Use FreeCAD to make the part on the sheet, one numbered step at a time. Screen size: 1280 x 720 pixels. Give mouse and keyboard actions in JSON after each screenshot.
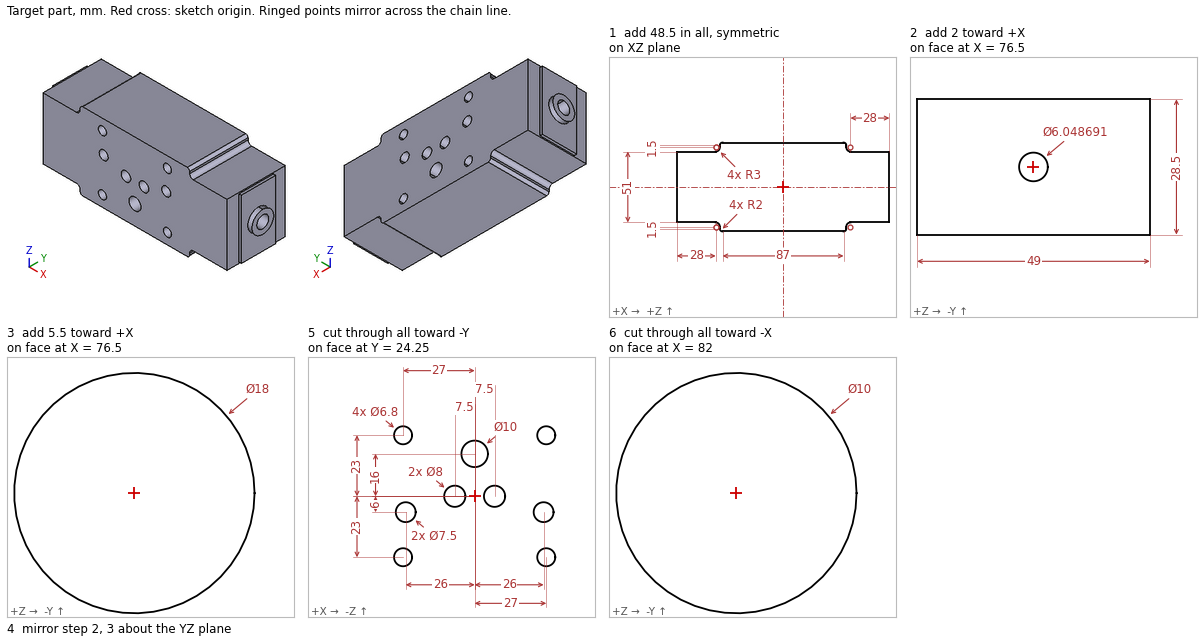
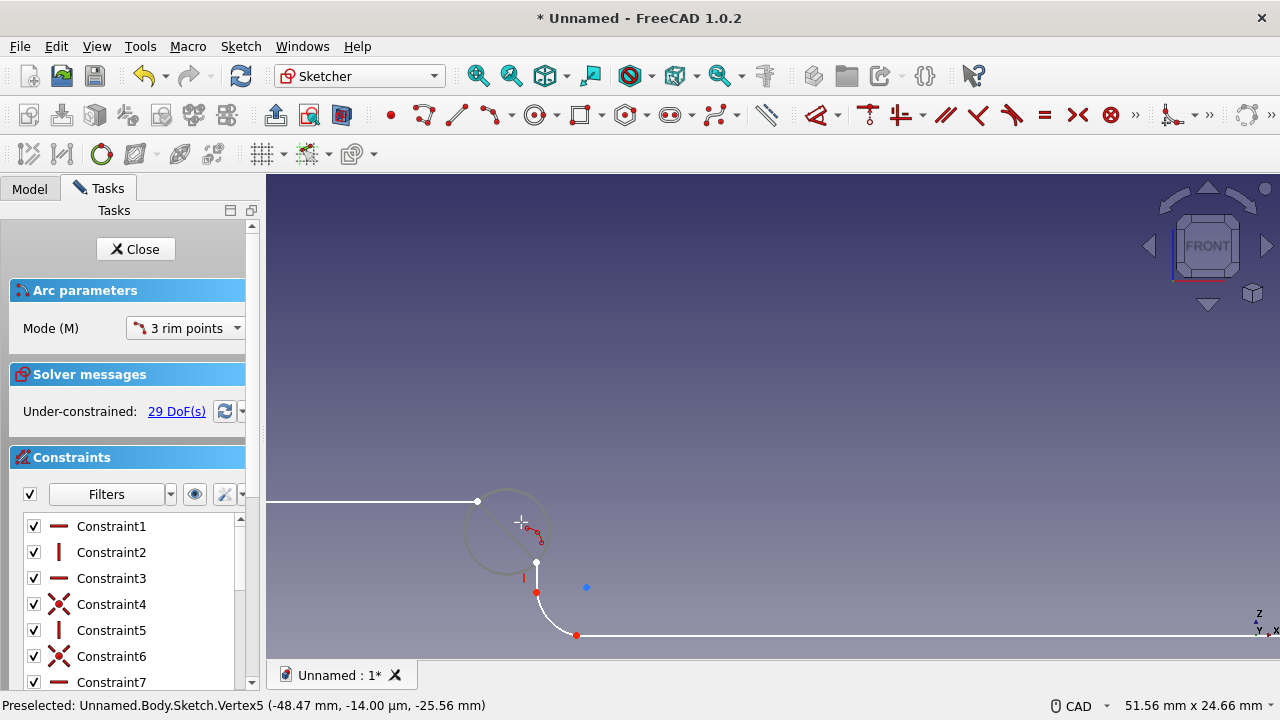
{"action": "left_click", "coordinate": [518, 518]}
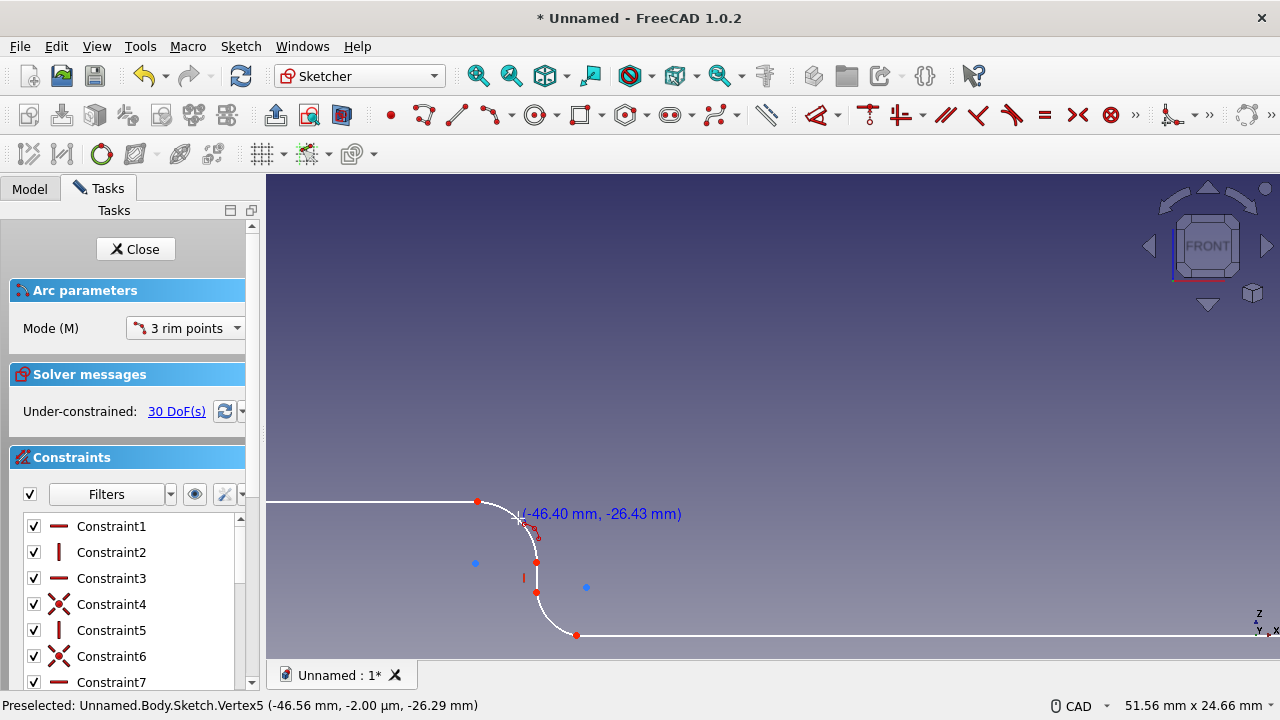
{"action": "scroll", "coordinate": [521, 522], "scroll_direction": "down", "scroll_amount": 8}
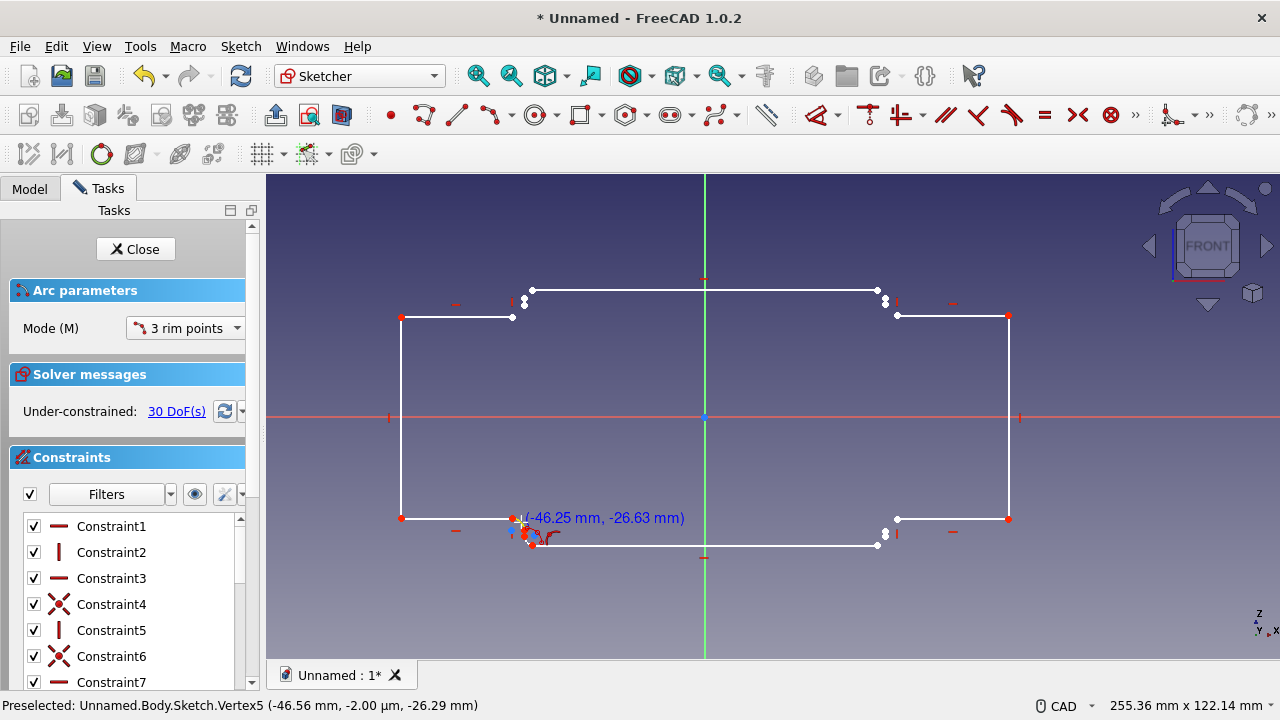
{"action": "left_click", "coordinate": [512, 317]}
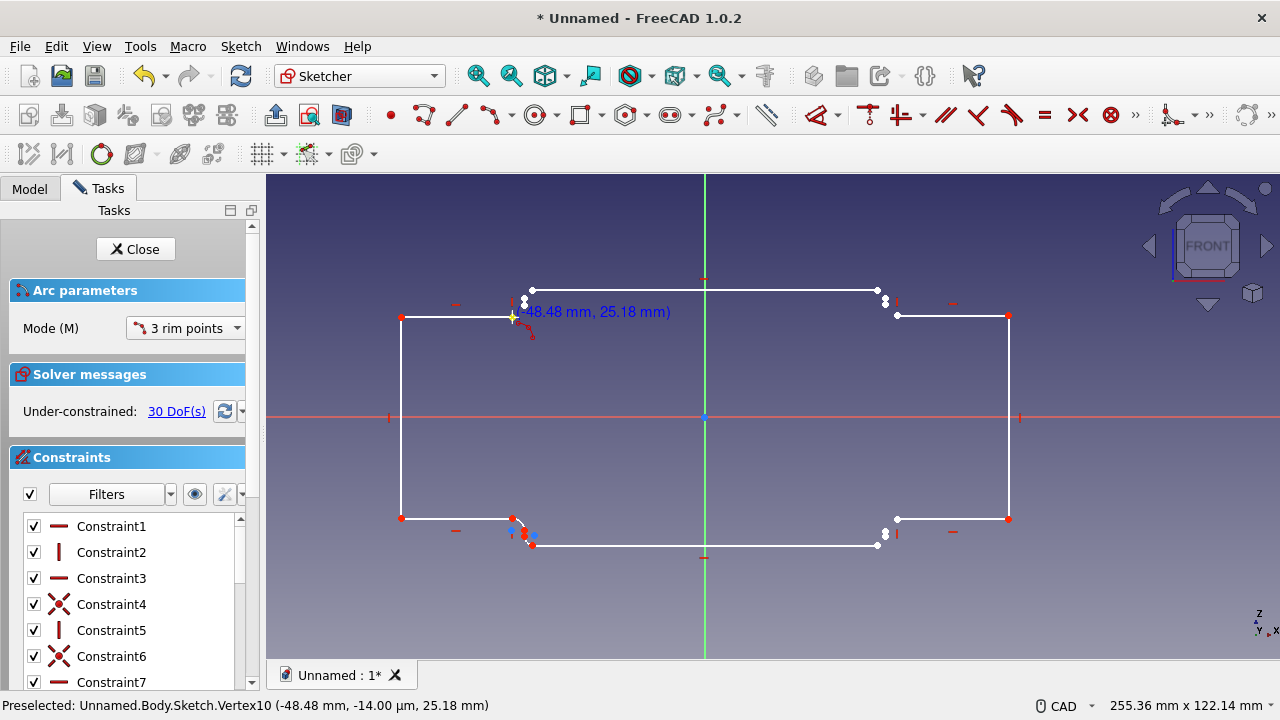
{"action": "scroll", "coordinate": [524, 304], "scroll_direction": "up", "scroll_amount": 9}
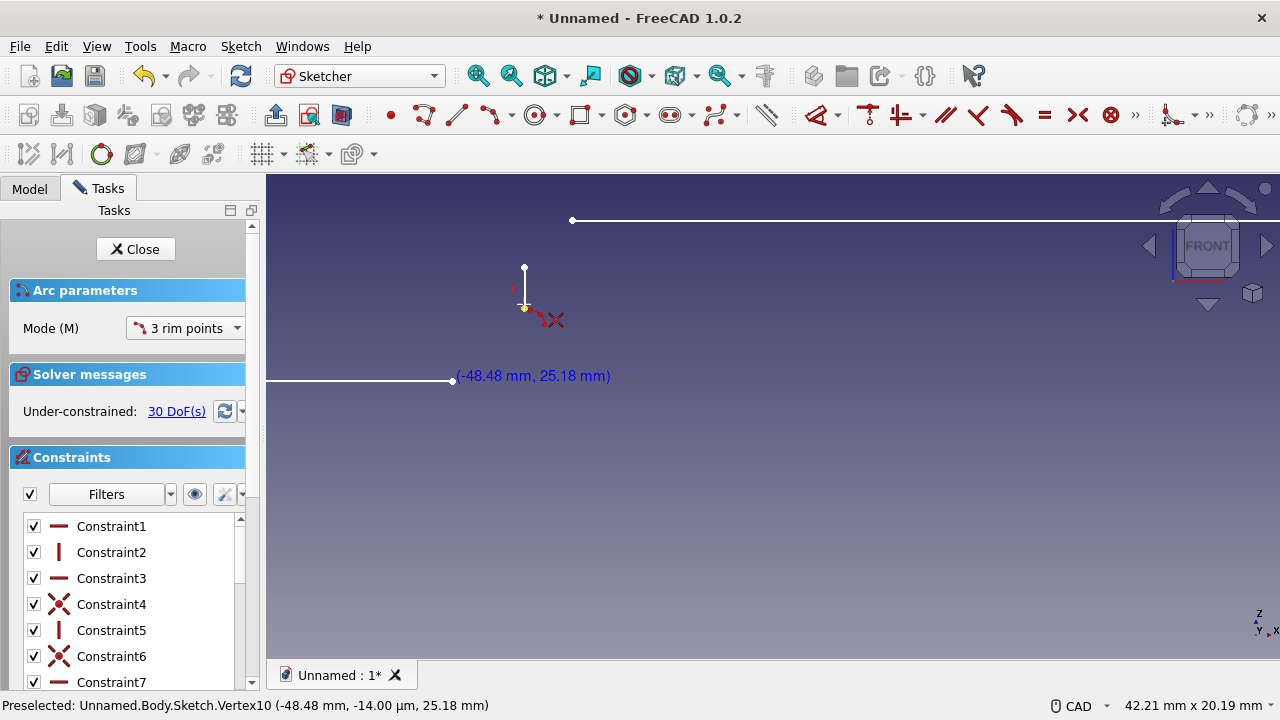
{"action": "left_click", "coordinate": [525, 309]}
{"action": "left_click", "coordinate": [503, 353]}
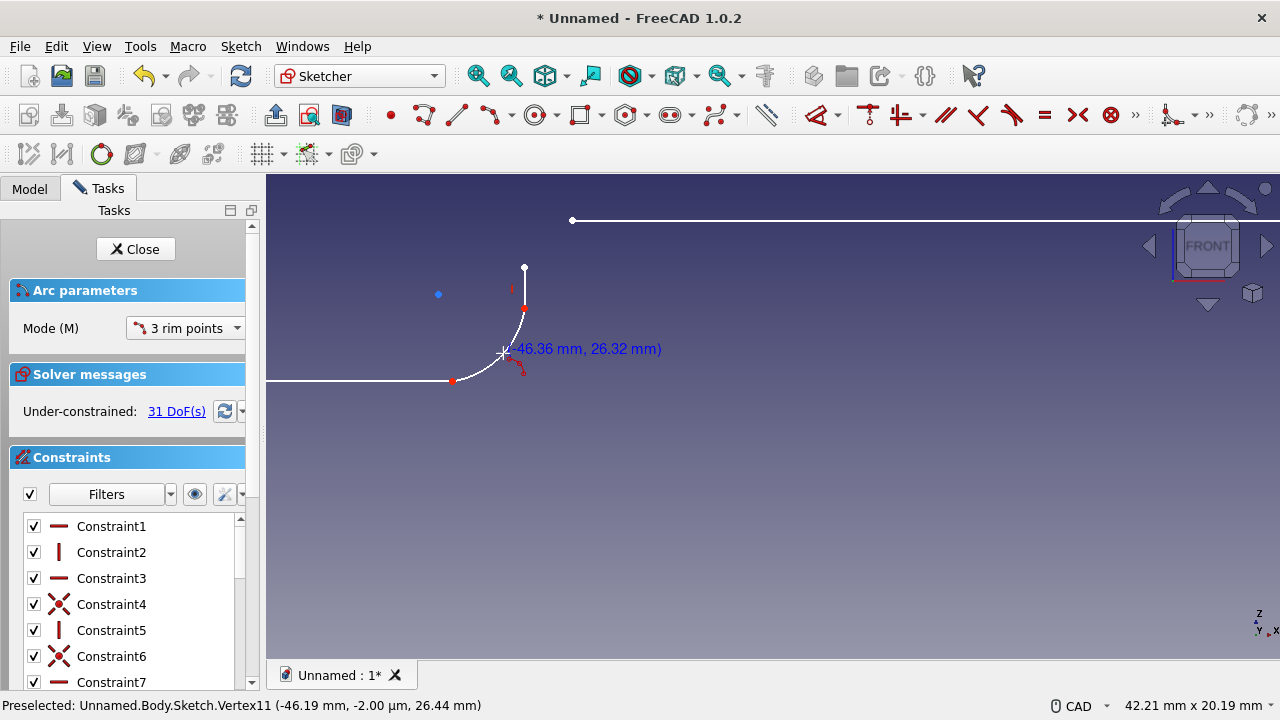
{"action": "left_click", "coordinate": [525, 267]}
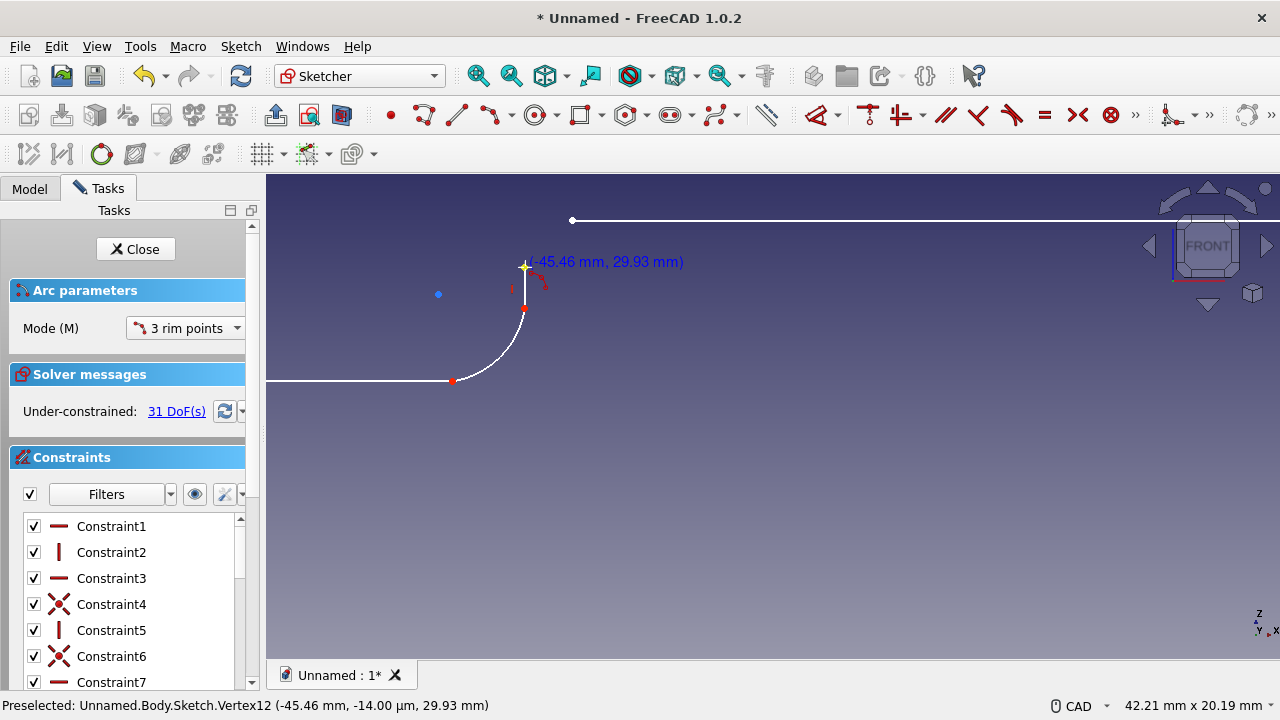
{"action": "scroll", "coordinate": [524, 304], "scroll_direction": "down", "scroll_amount": 9}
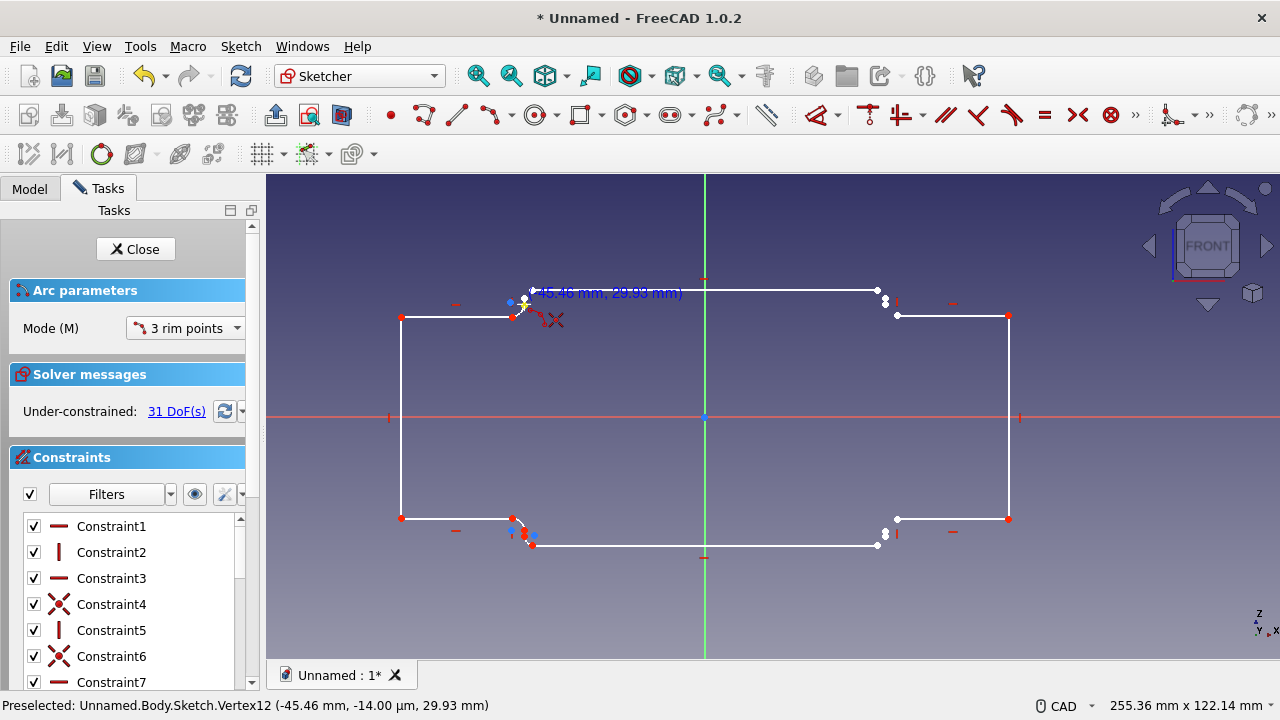
{"action": "scroll", "coordinate": [532, 290], "scroll_direction": "up", "scroll_amount": 2}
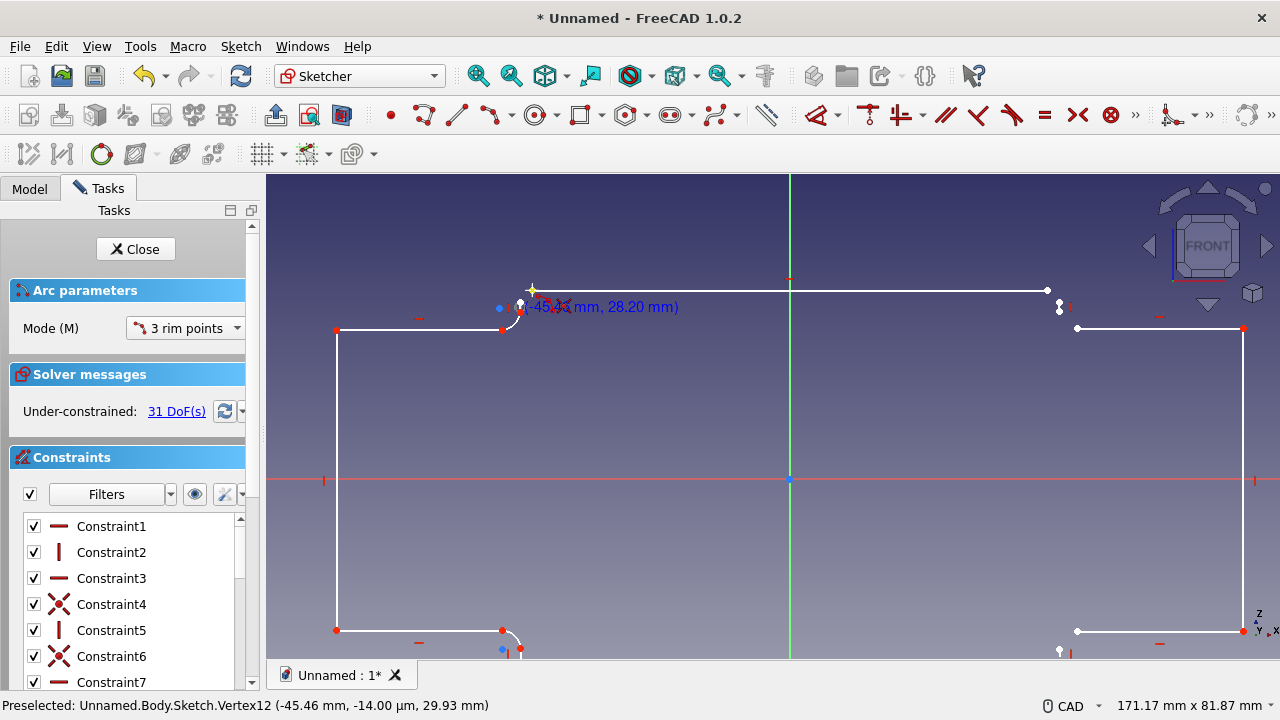
{"action": "left_click", "coordinate": [532, 291]}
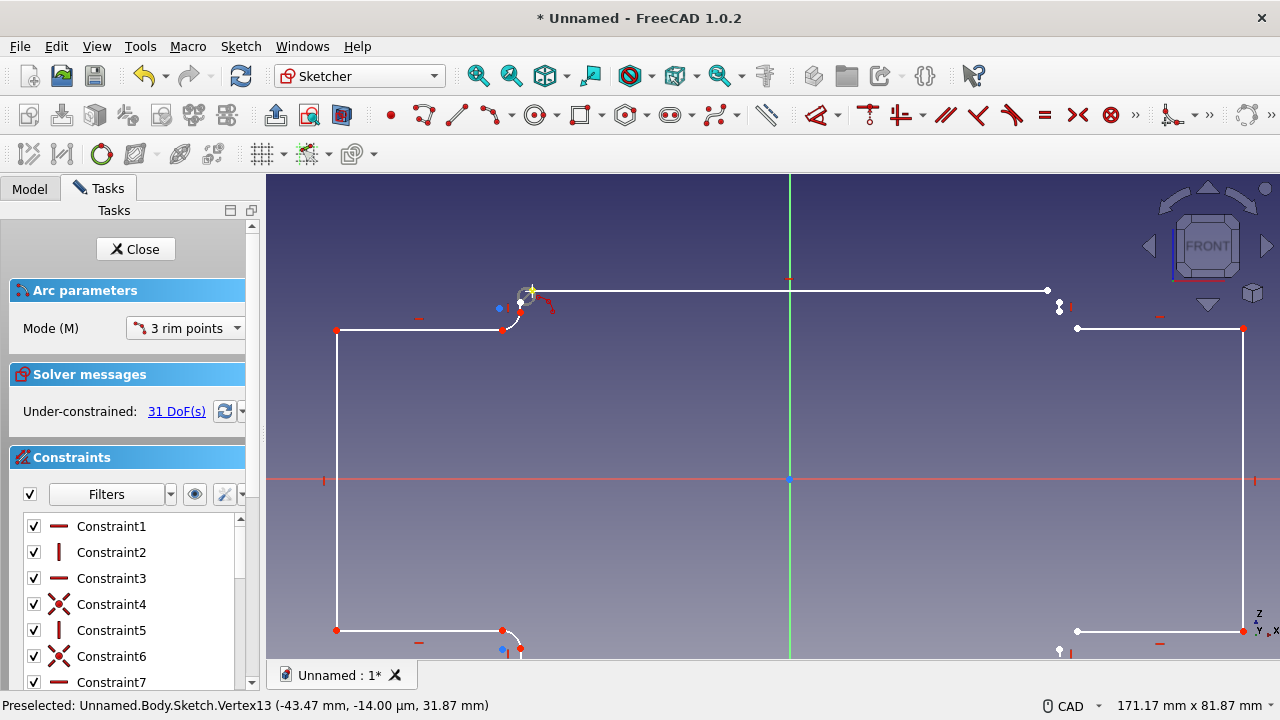
{"action": "scroll", "coordinate": [524, 293], "scroll_direction": "up", "scroll_amount": 8}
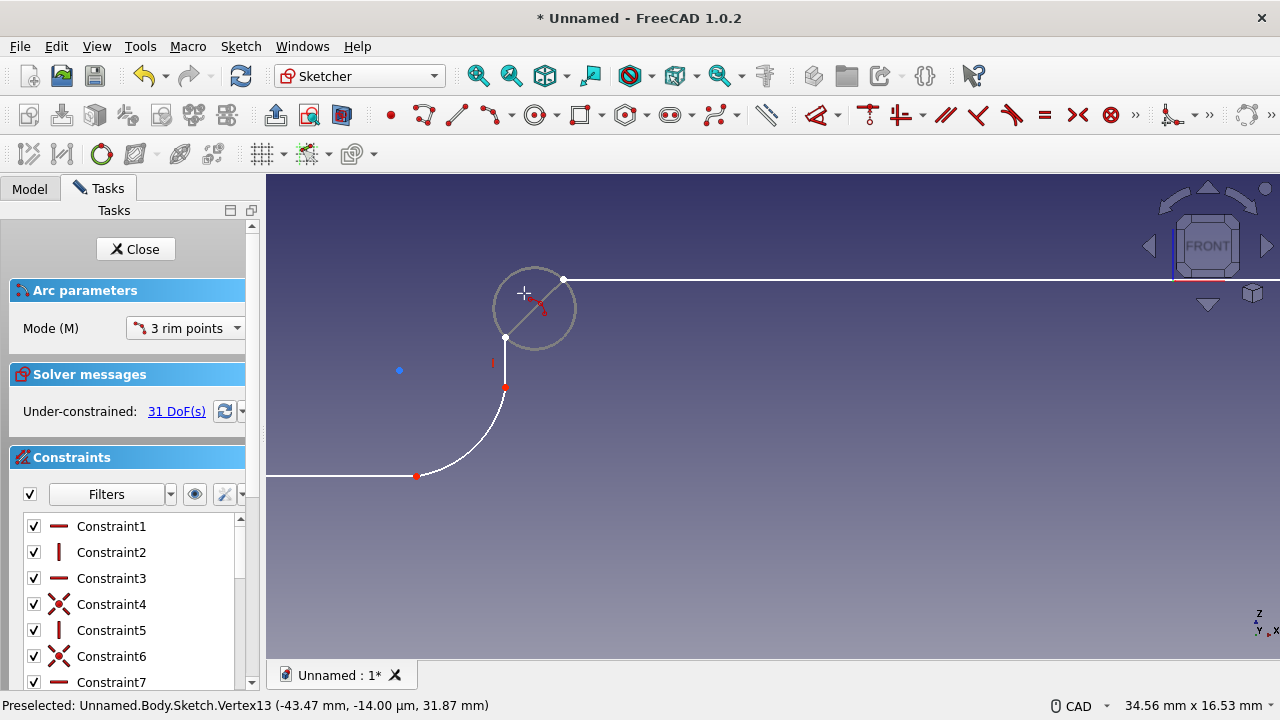
{"action": "left_click", "coordinate": [521, 293]}